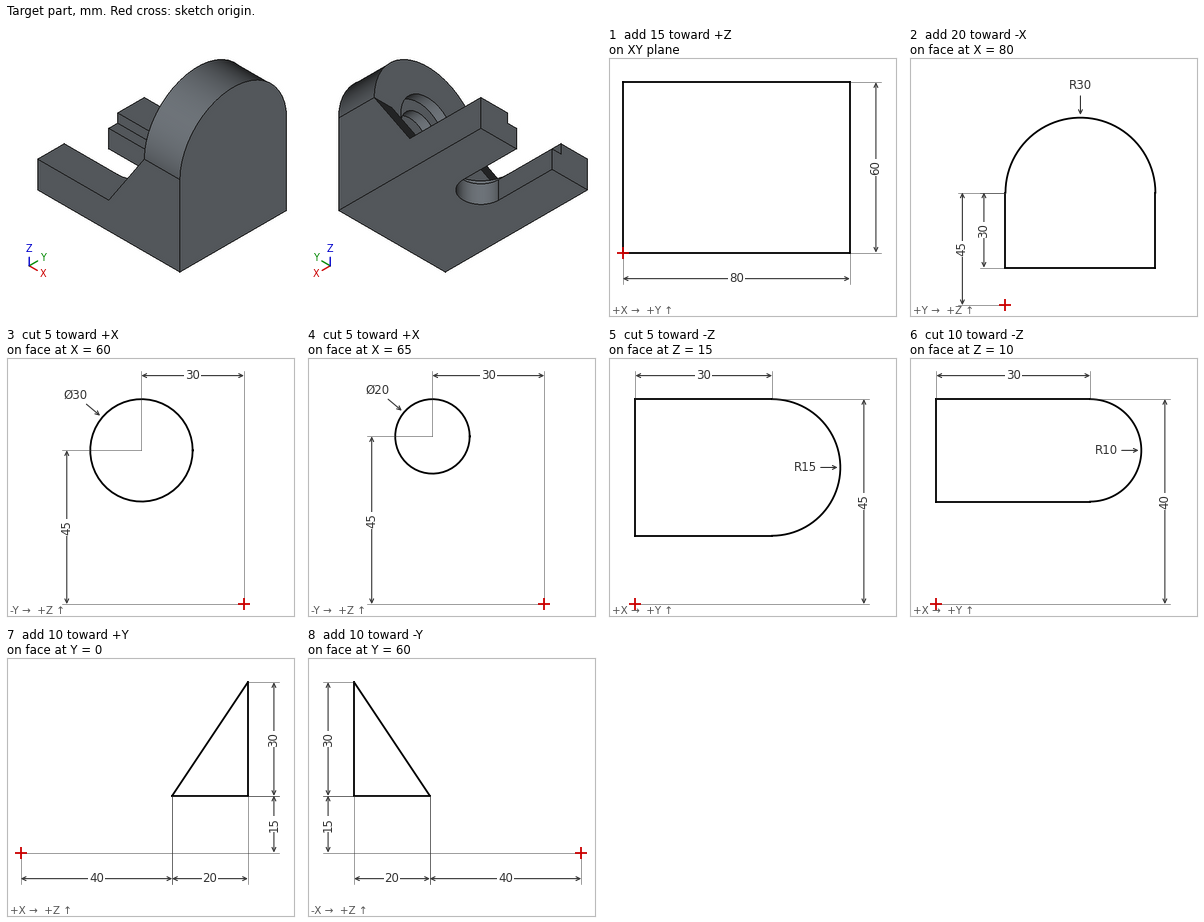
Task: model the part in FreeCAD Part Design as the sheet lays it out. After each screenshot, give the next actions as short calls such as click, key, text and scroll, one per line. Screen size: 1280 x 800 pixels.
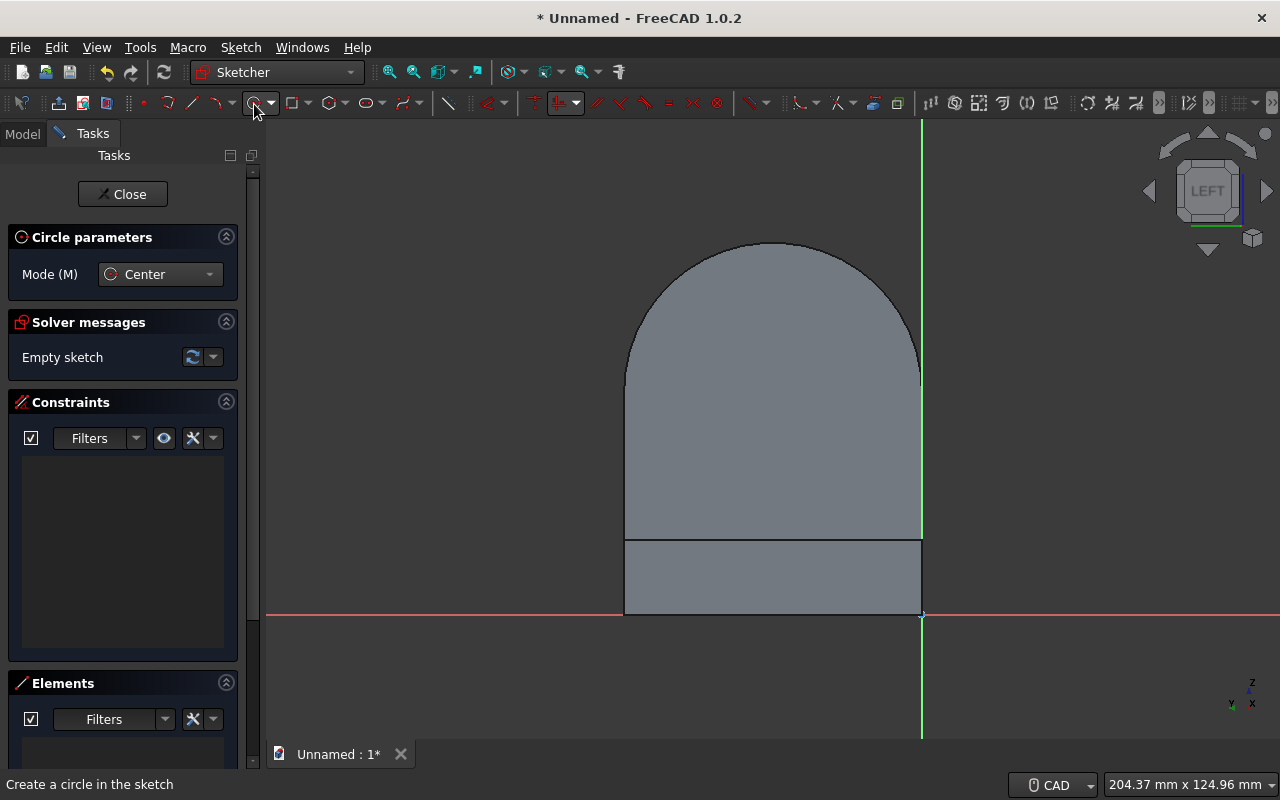
click(773, 392)
click(826, 339)
key(Escape)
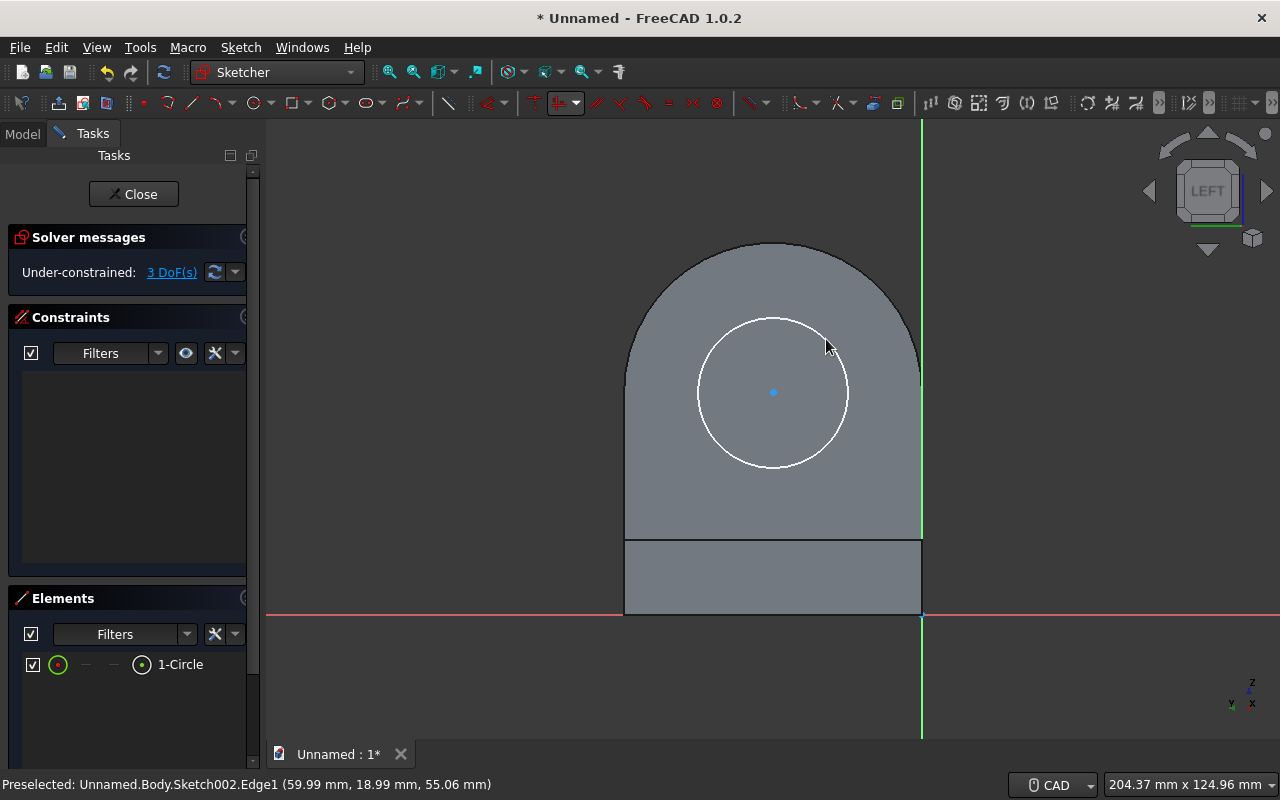
click(488, 104)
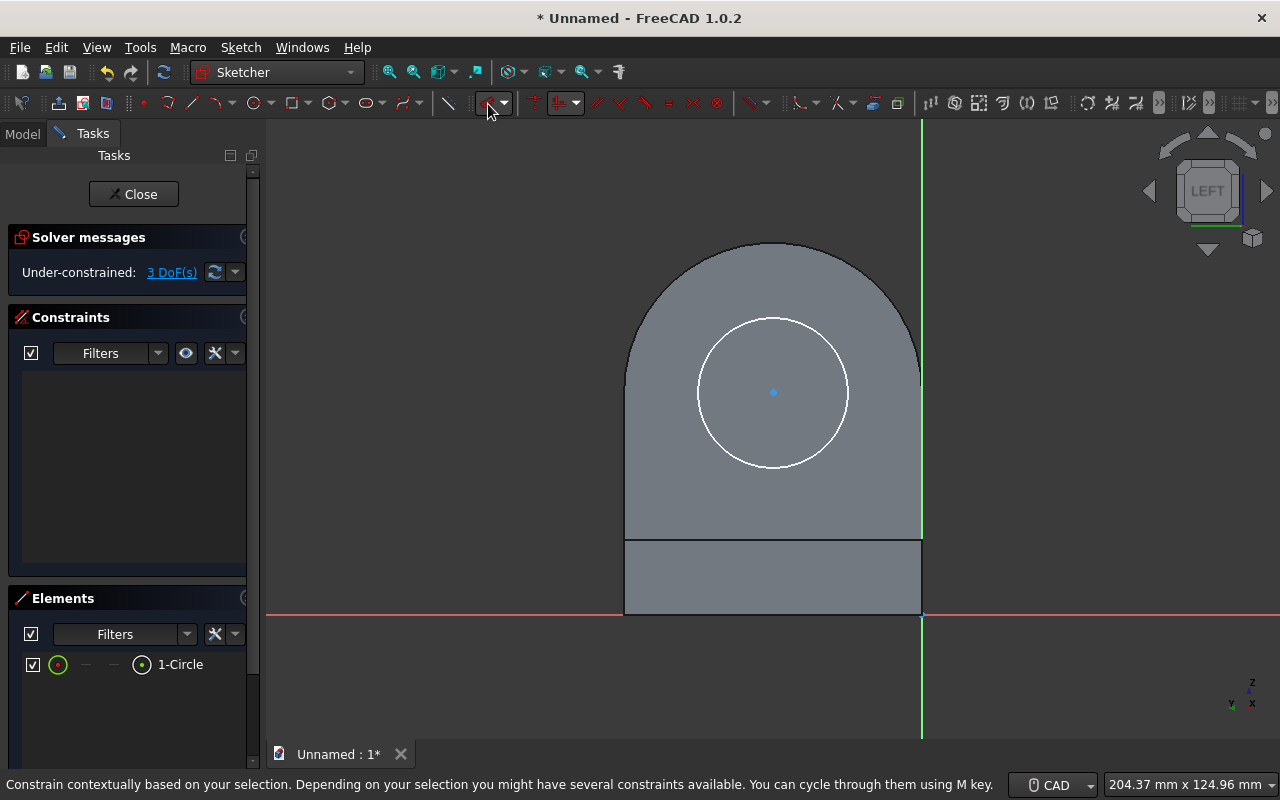
click(826, 340)
click(849, 317)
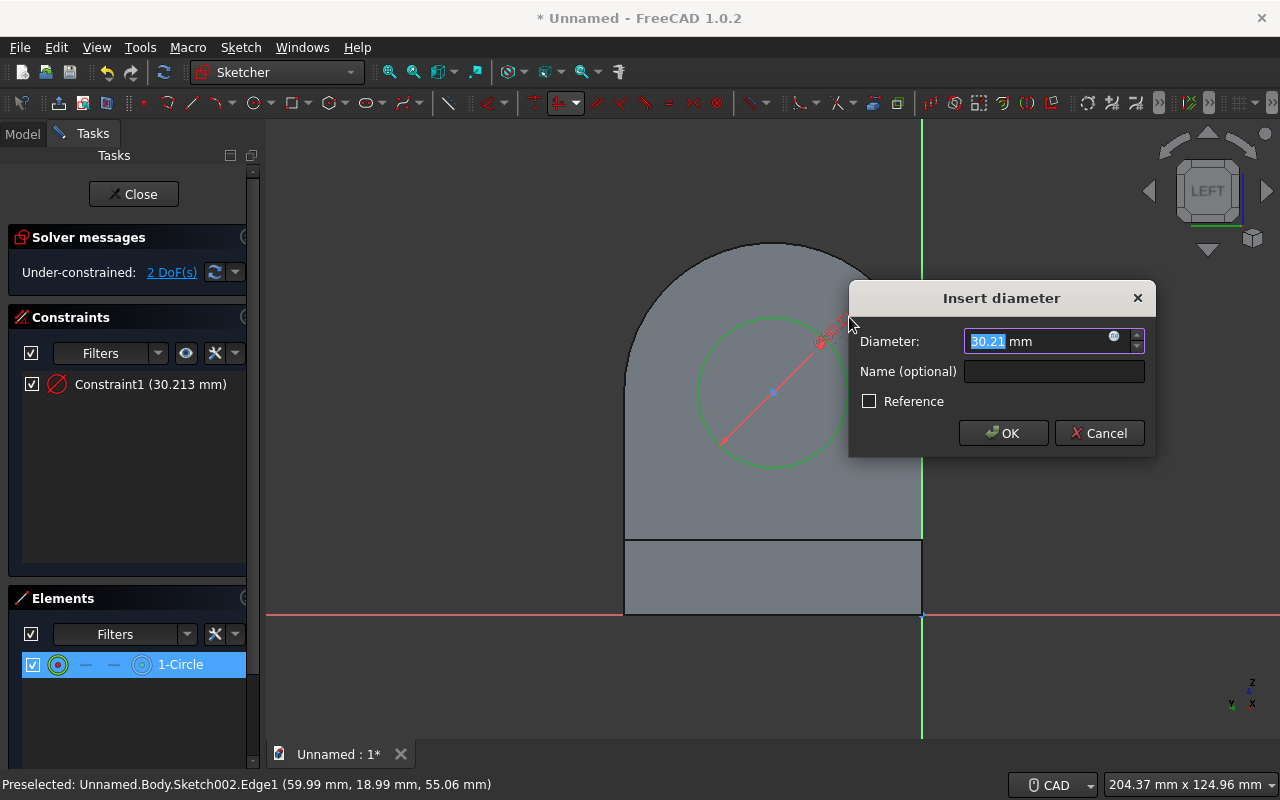
text(30)
key(Return)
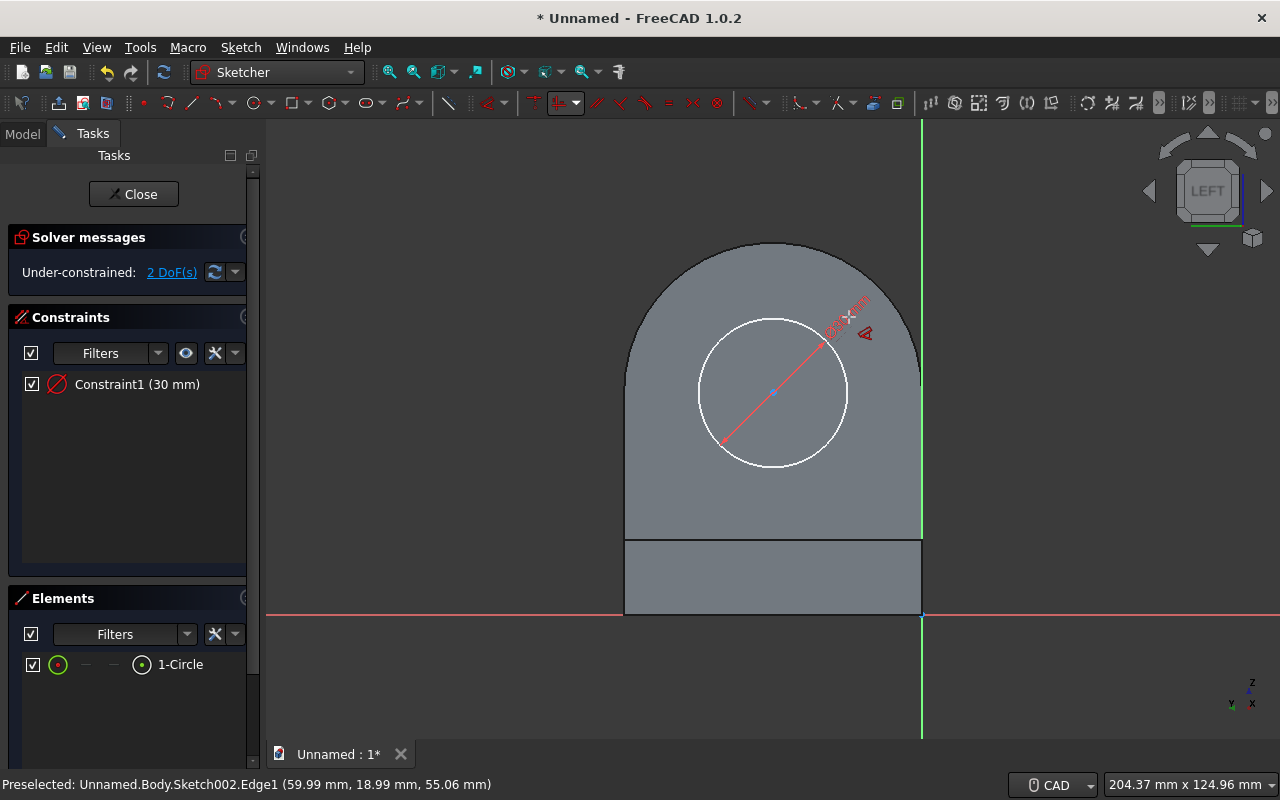
click(773, 393)
click(847, 649)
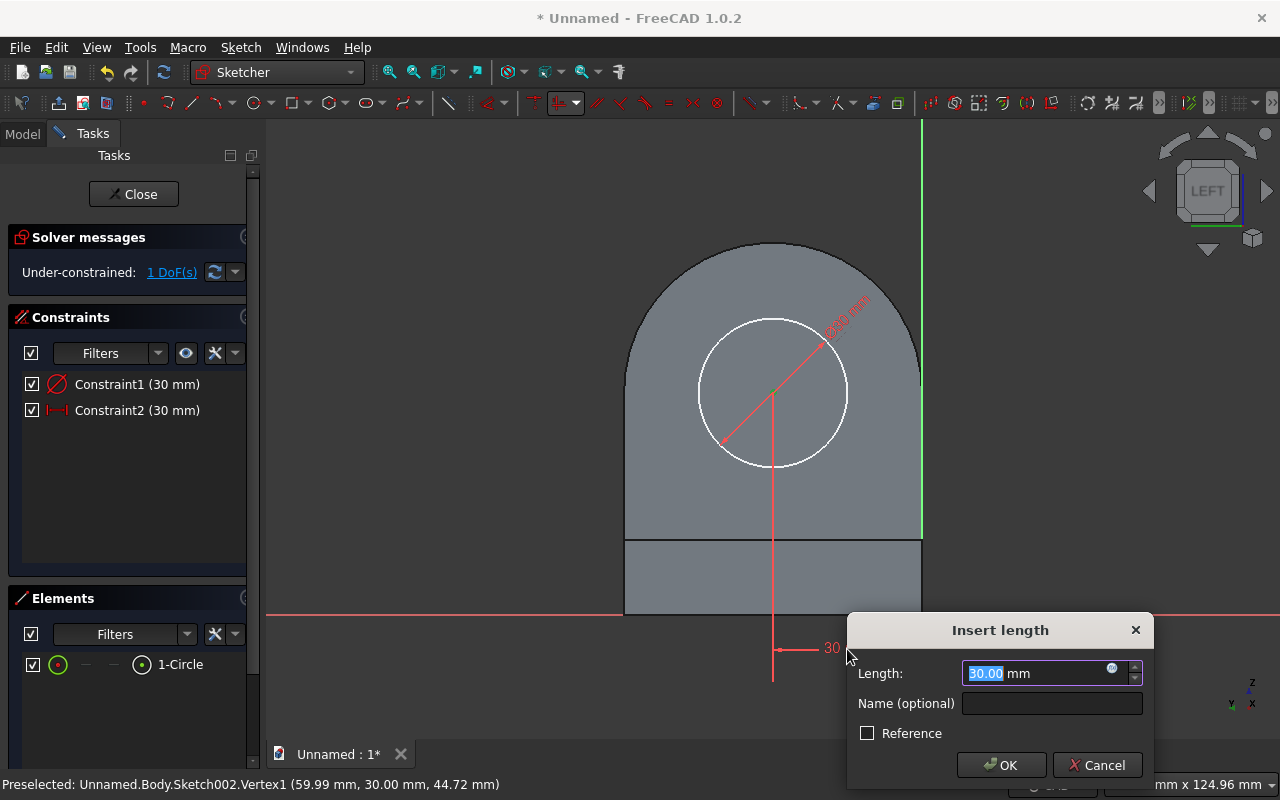
text(30)
key(Return)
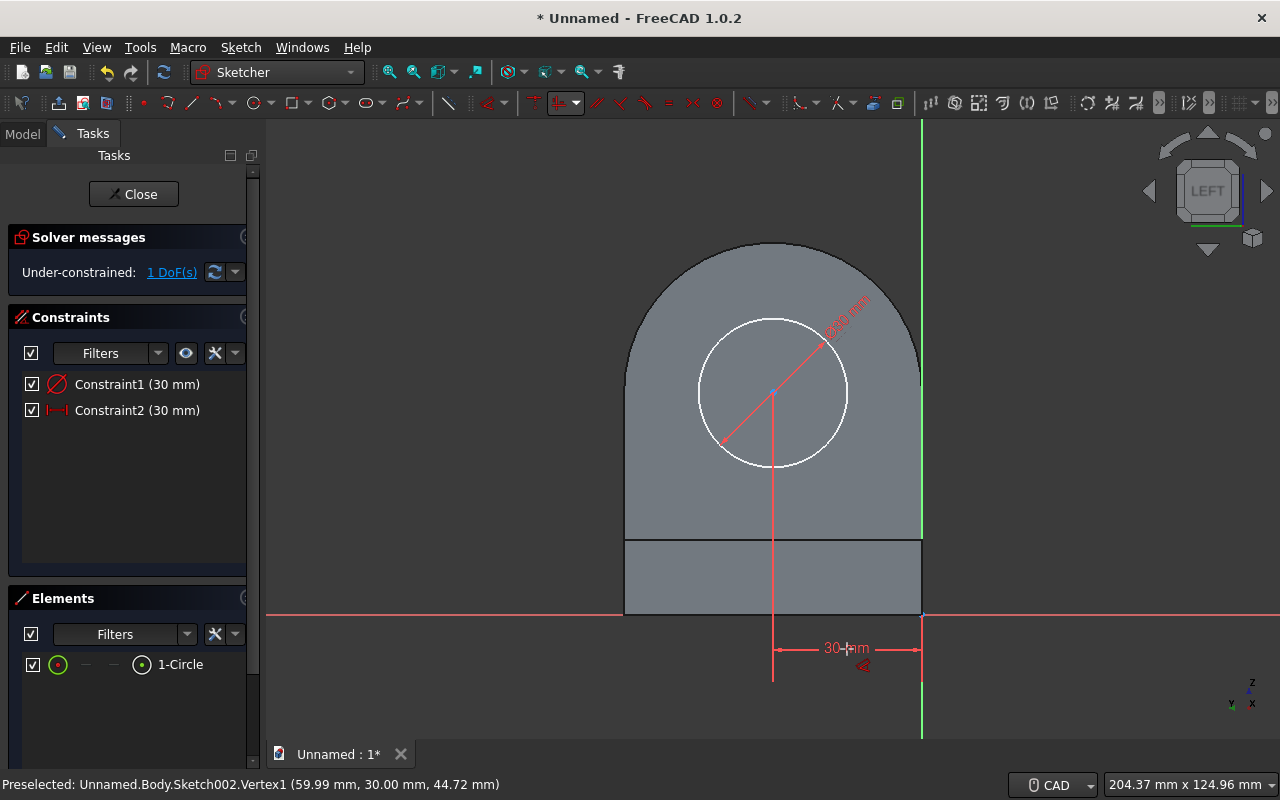
click(773, 393)
click(956, 504)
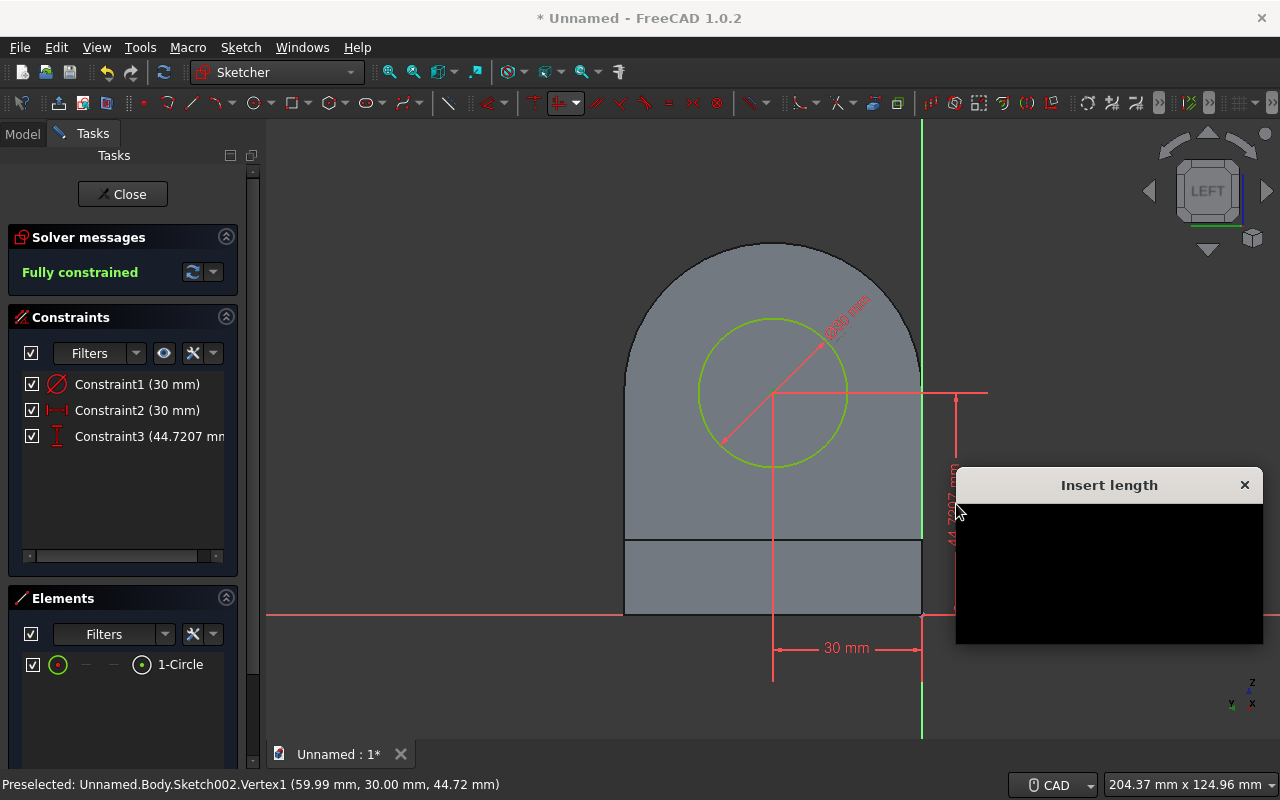
text(45)
key(Return)
key(Escape)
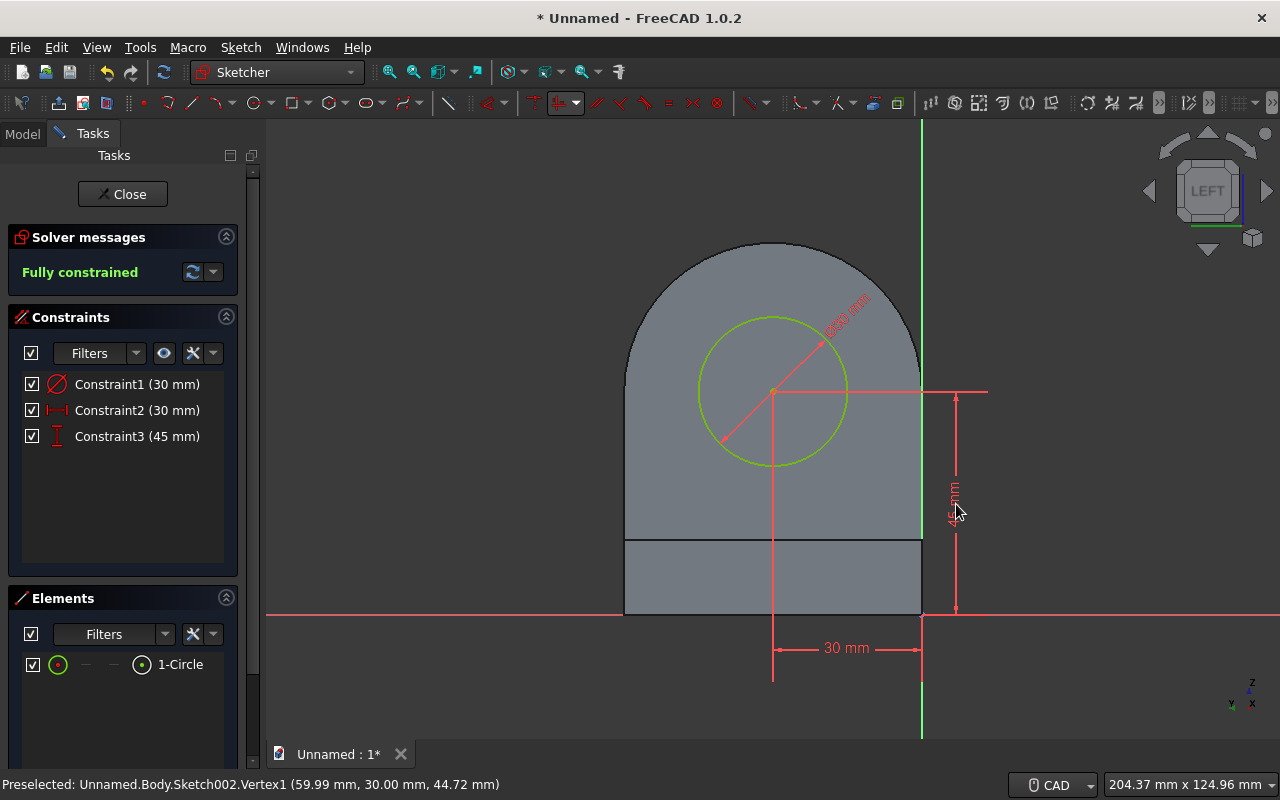
click(123, 194)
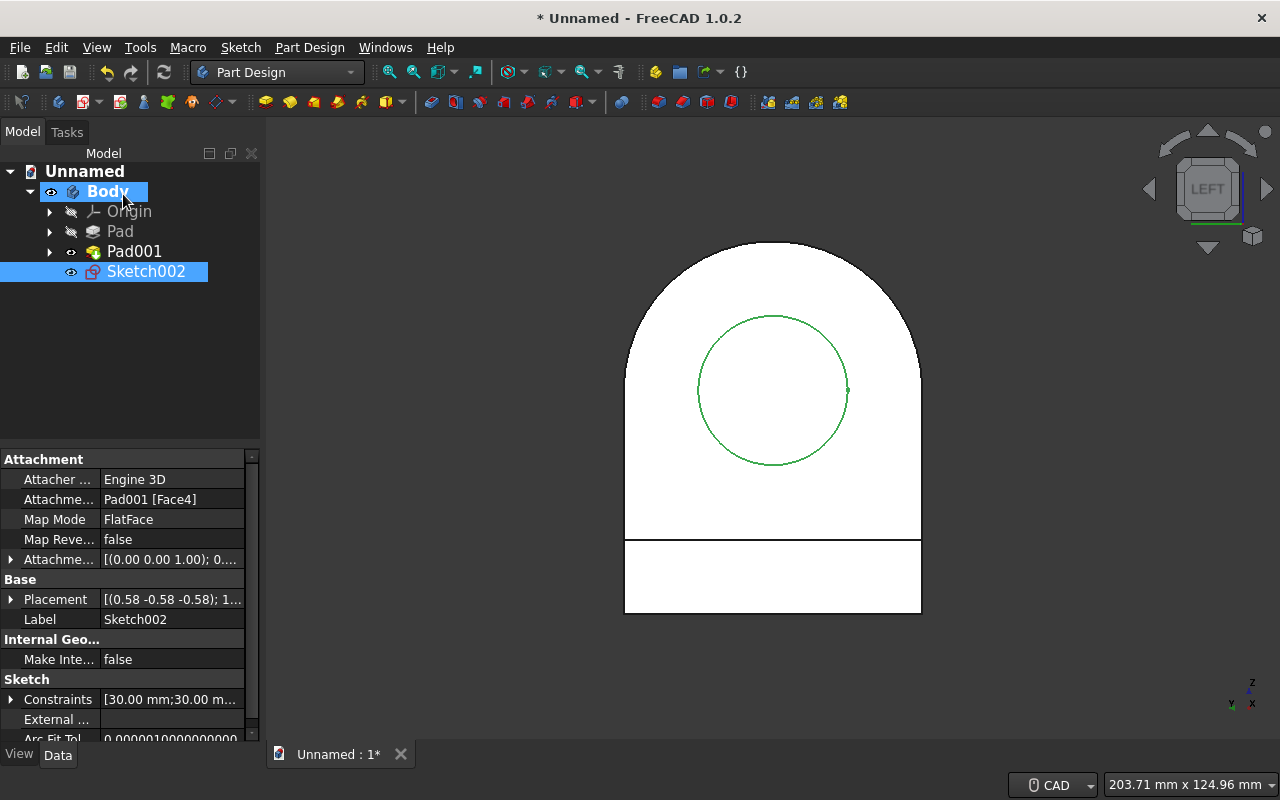
click(432, 102)